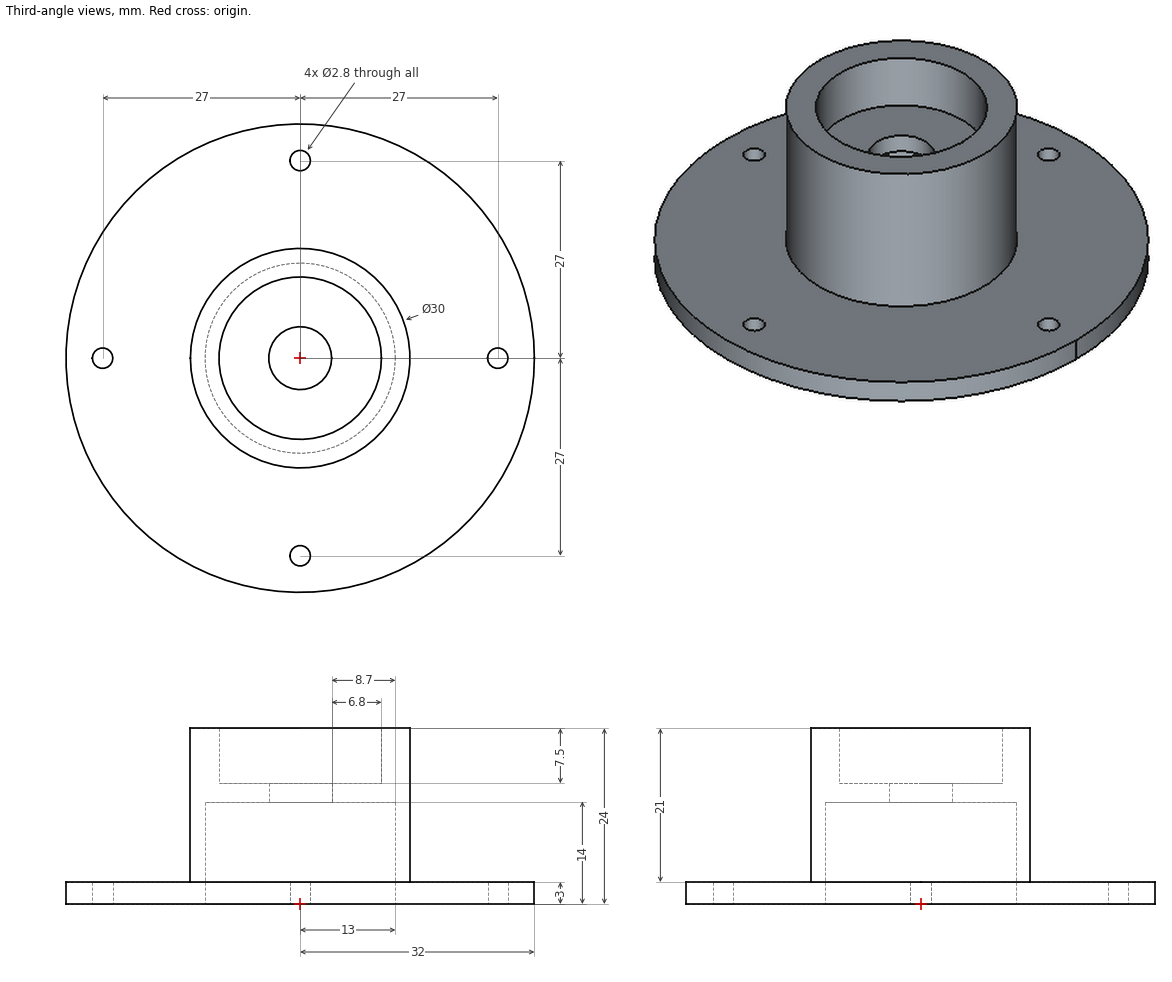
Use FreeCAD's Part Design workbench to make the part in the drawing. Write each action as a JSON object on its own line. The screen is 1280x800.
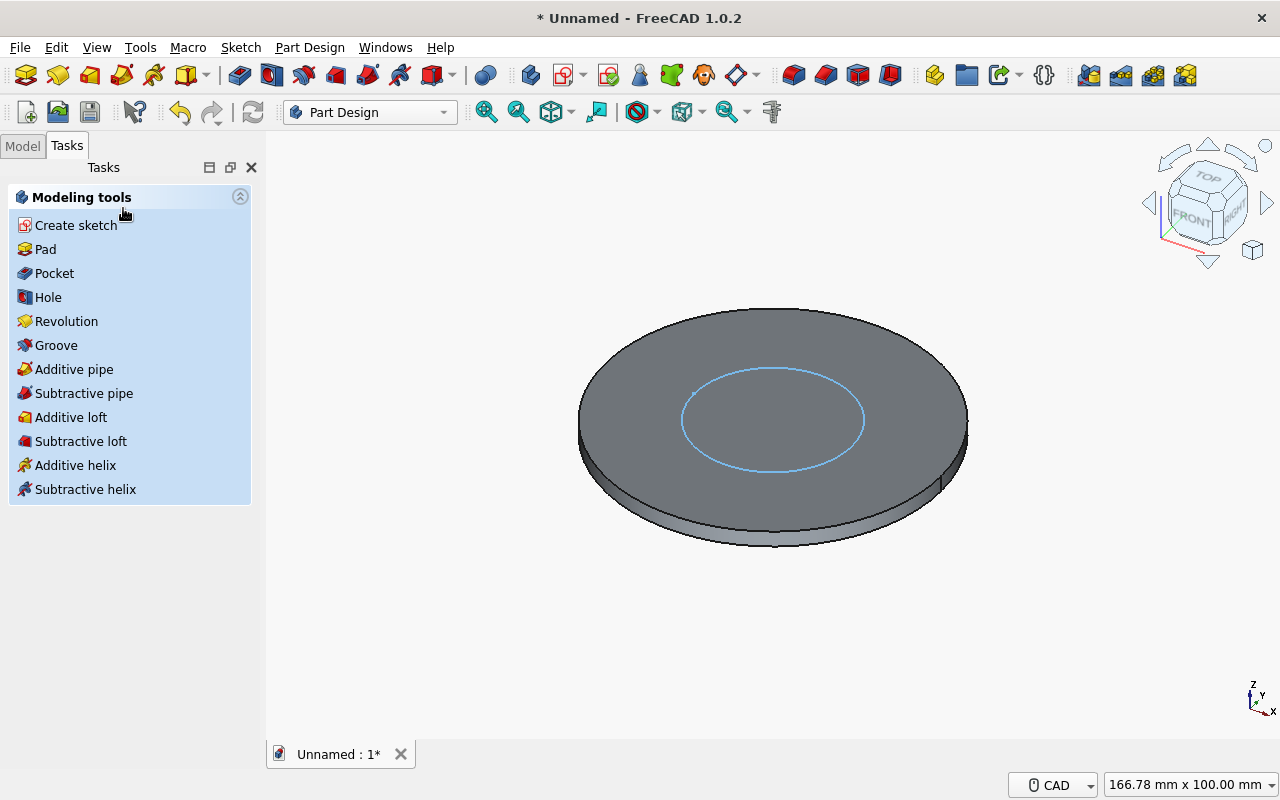
{"action": "left_click", "coordinate": [26, 76]}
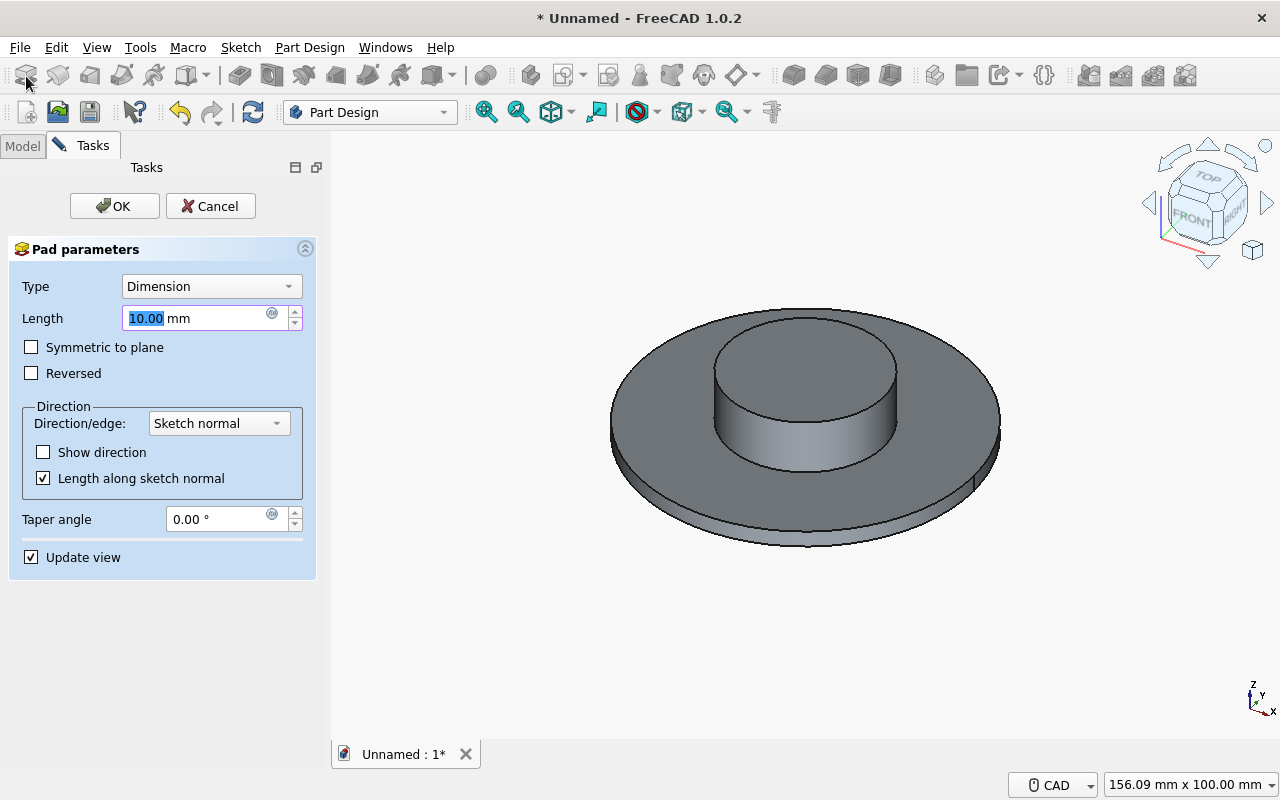
{"action": "type", "text": "21"}
{"action": "key", "text": "Tab"}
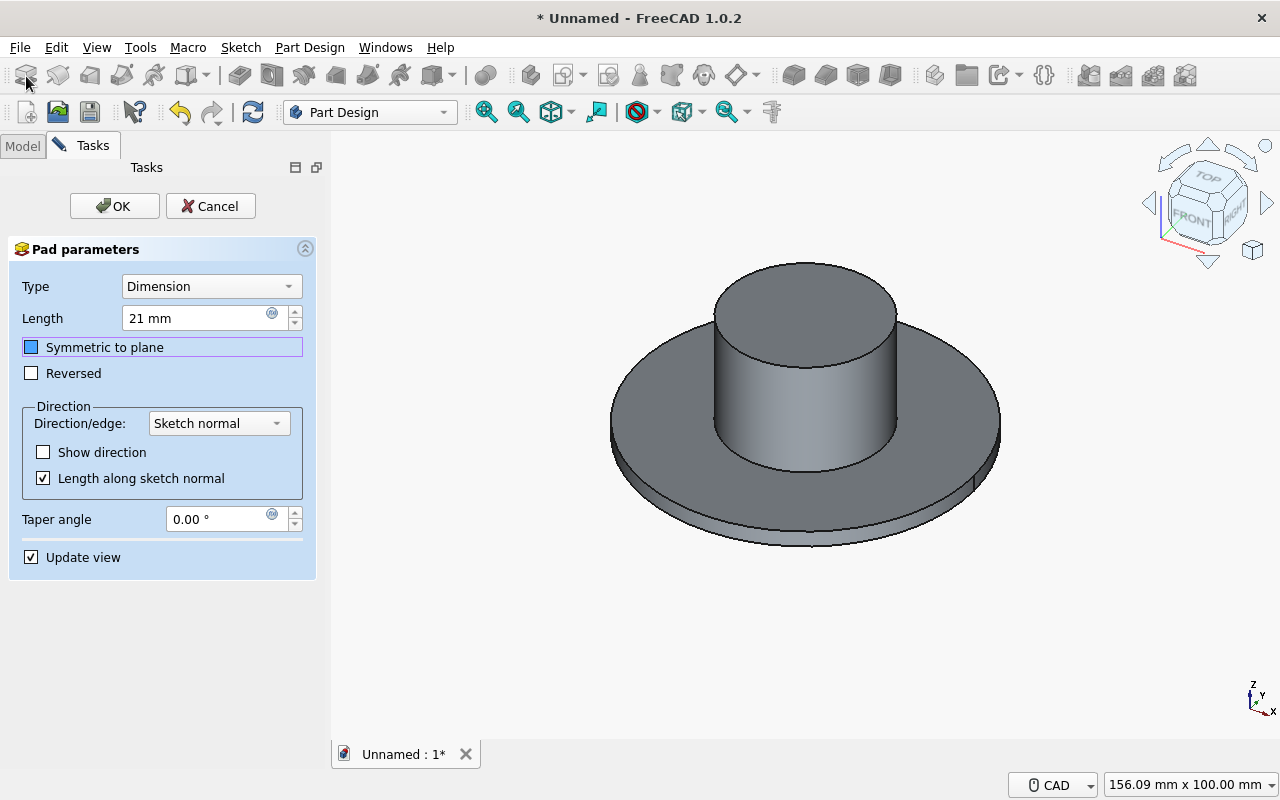
{"action": "left_click", "coordinate": [115, 206]}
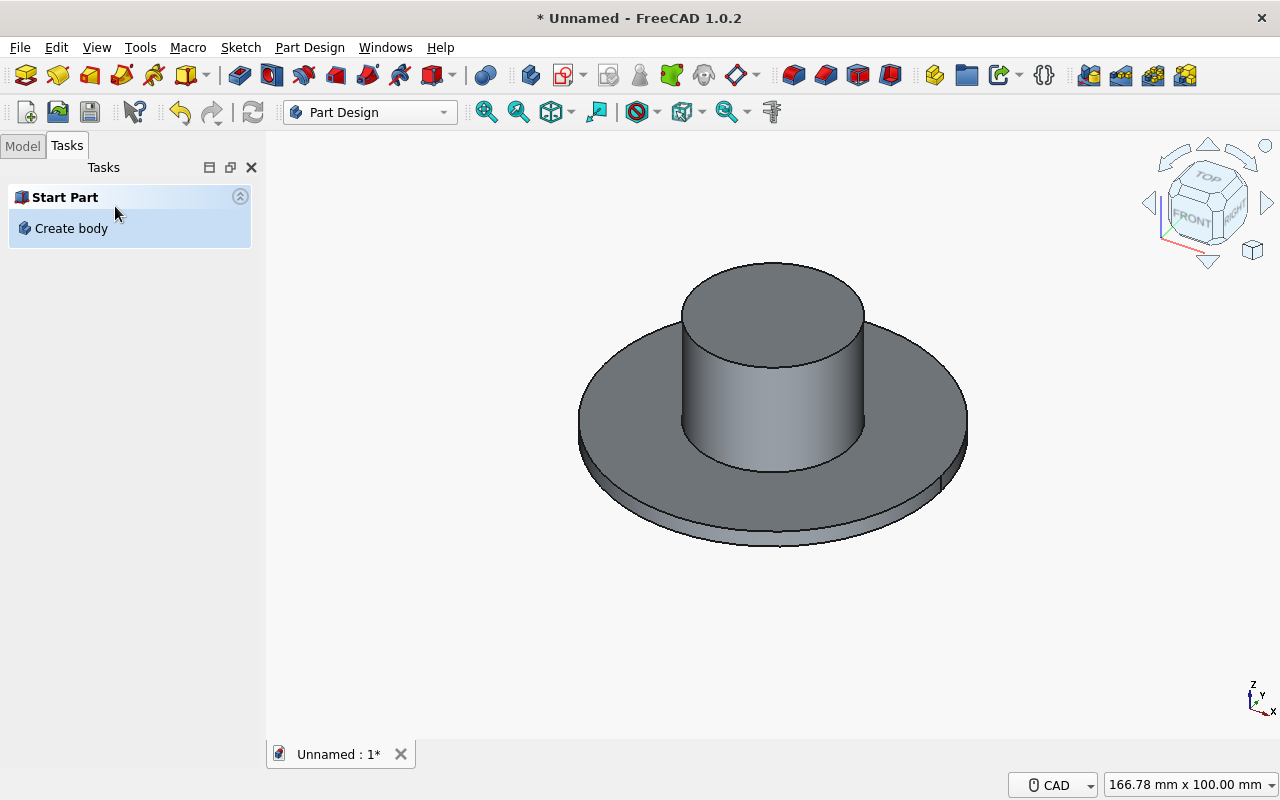
{"action": "left_click", "coordinate": [564, 76]}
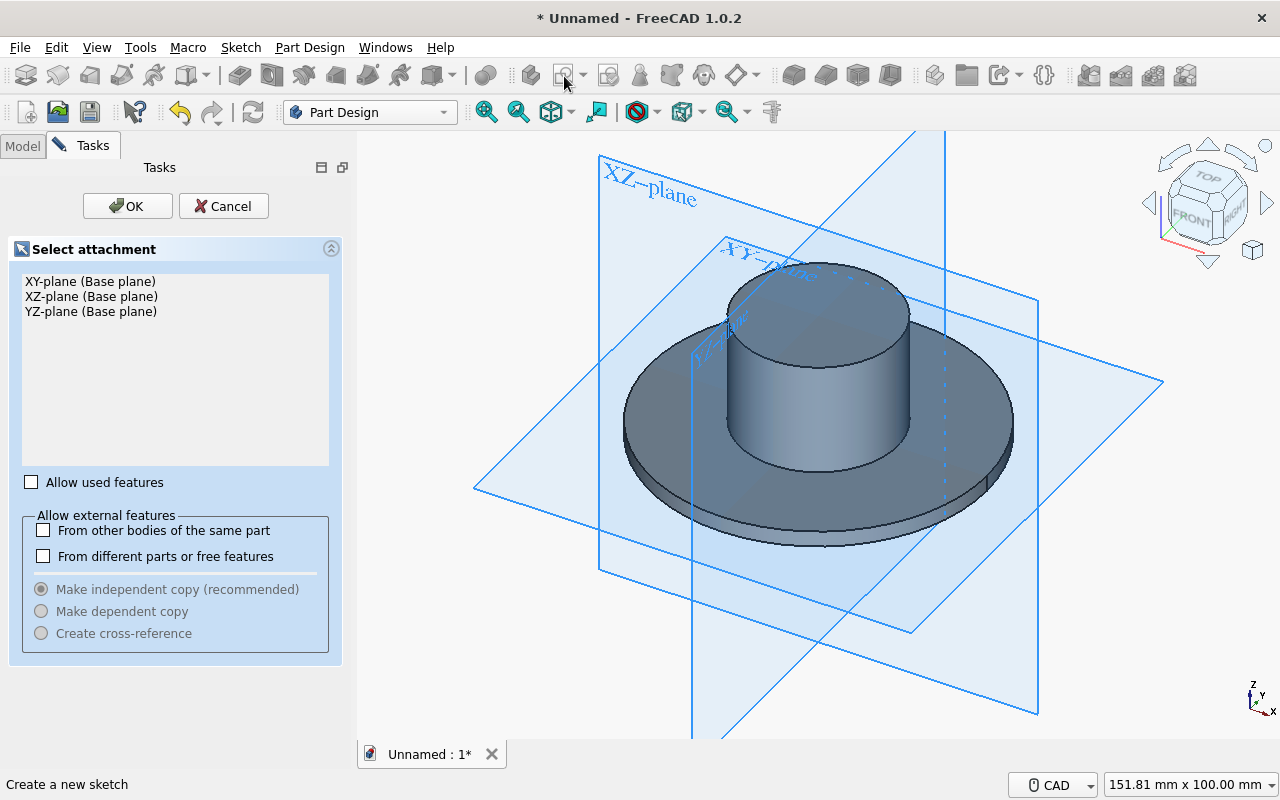
{"action": "left_click", "coordinate": [82, 296]}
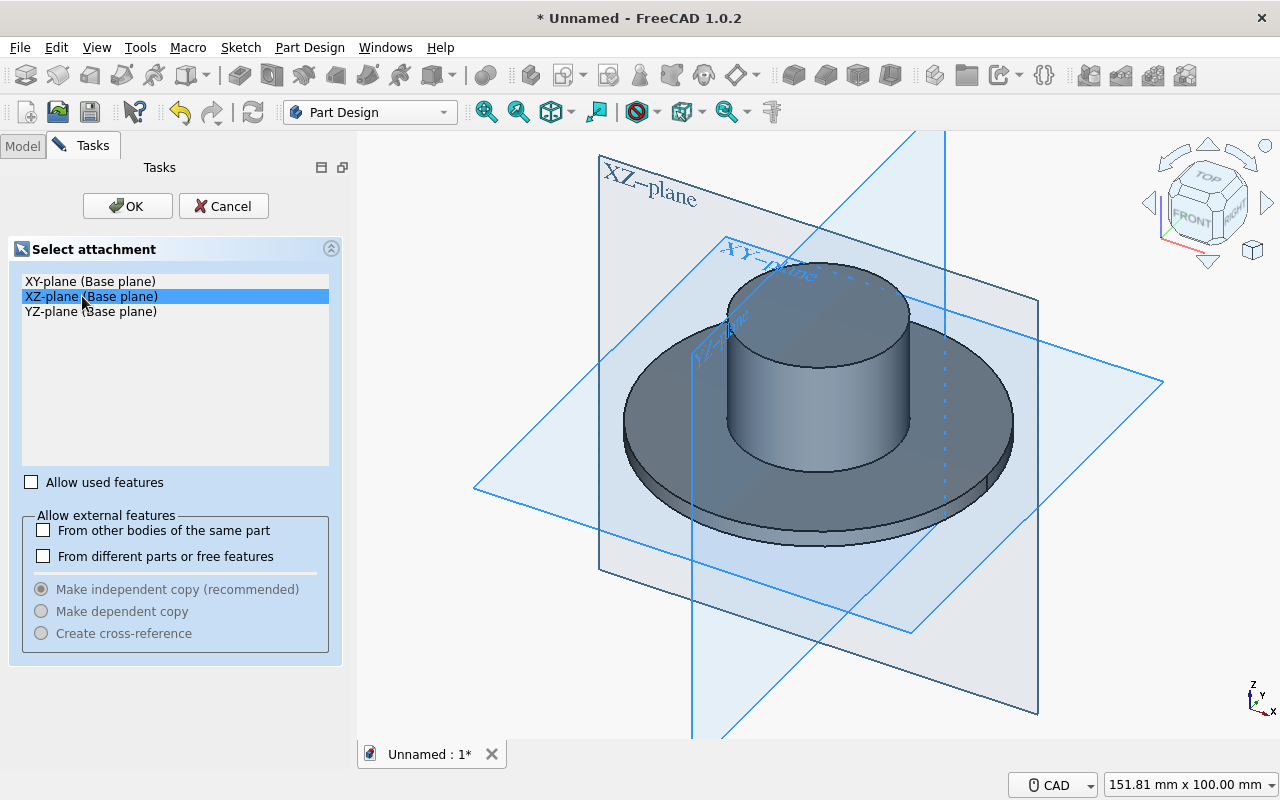
{"action": "left_click", "coordinate": [128, 206]}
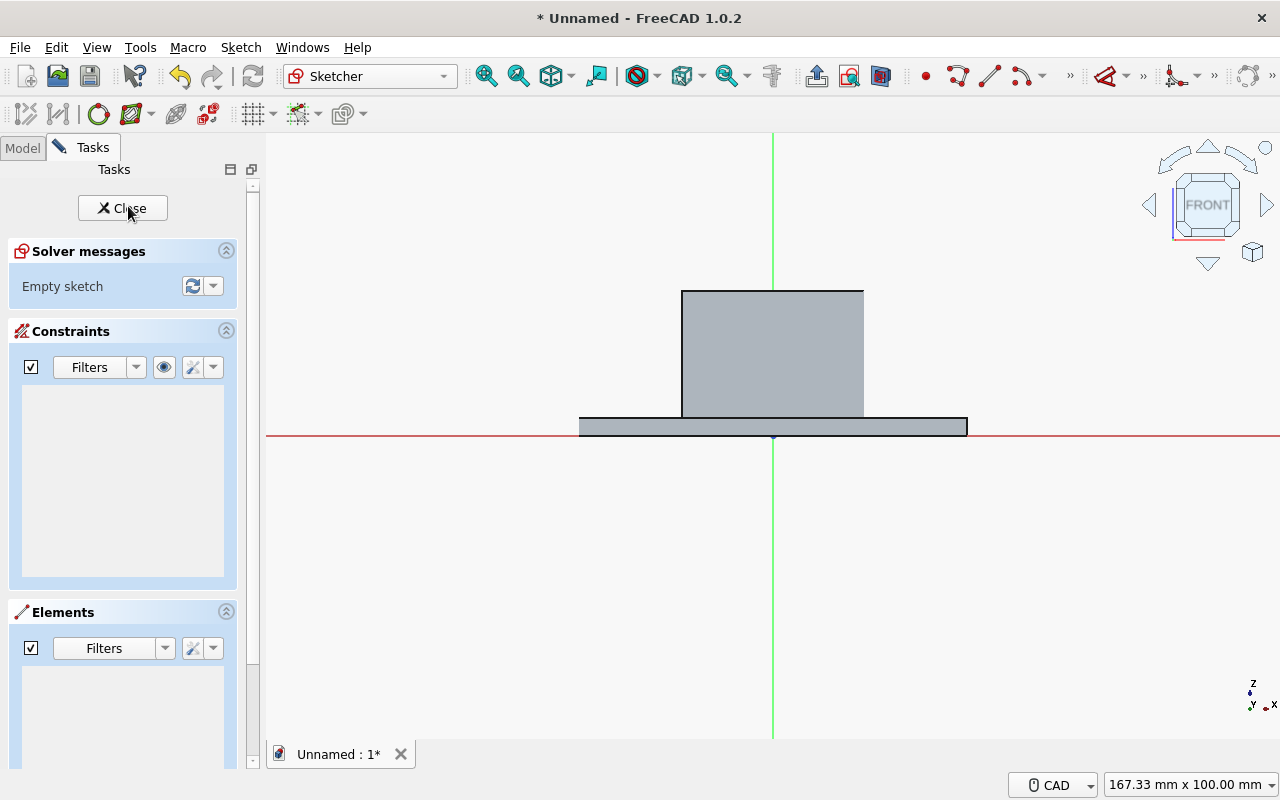
{"action": "left_click", "coordinate": [882, 76]}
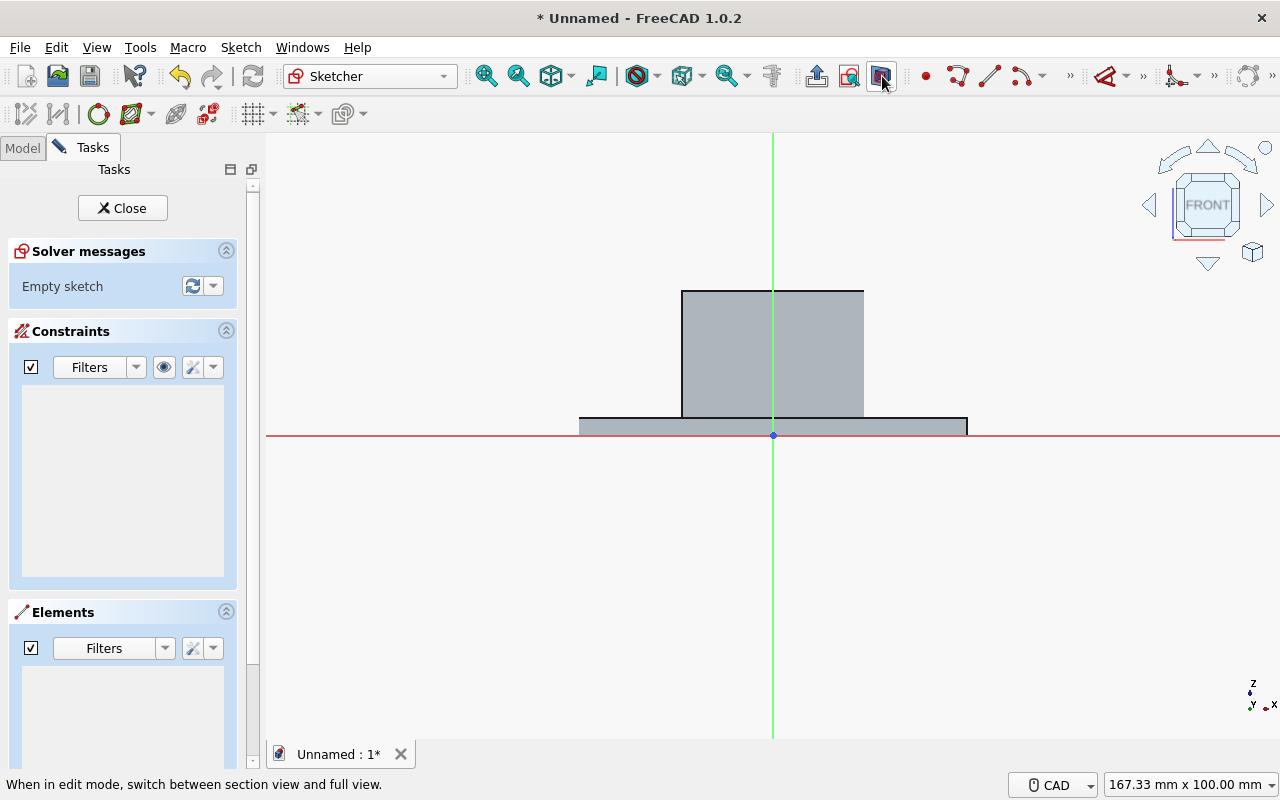
{"action": "scroll", "coordinate": [875, 321], "scroll_direction": "up", "scroll_amount": 5}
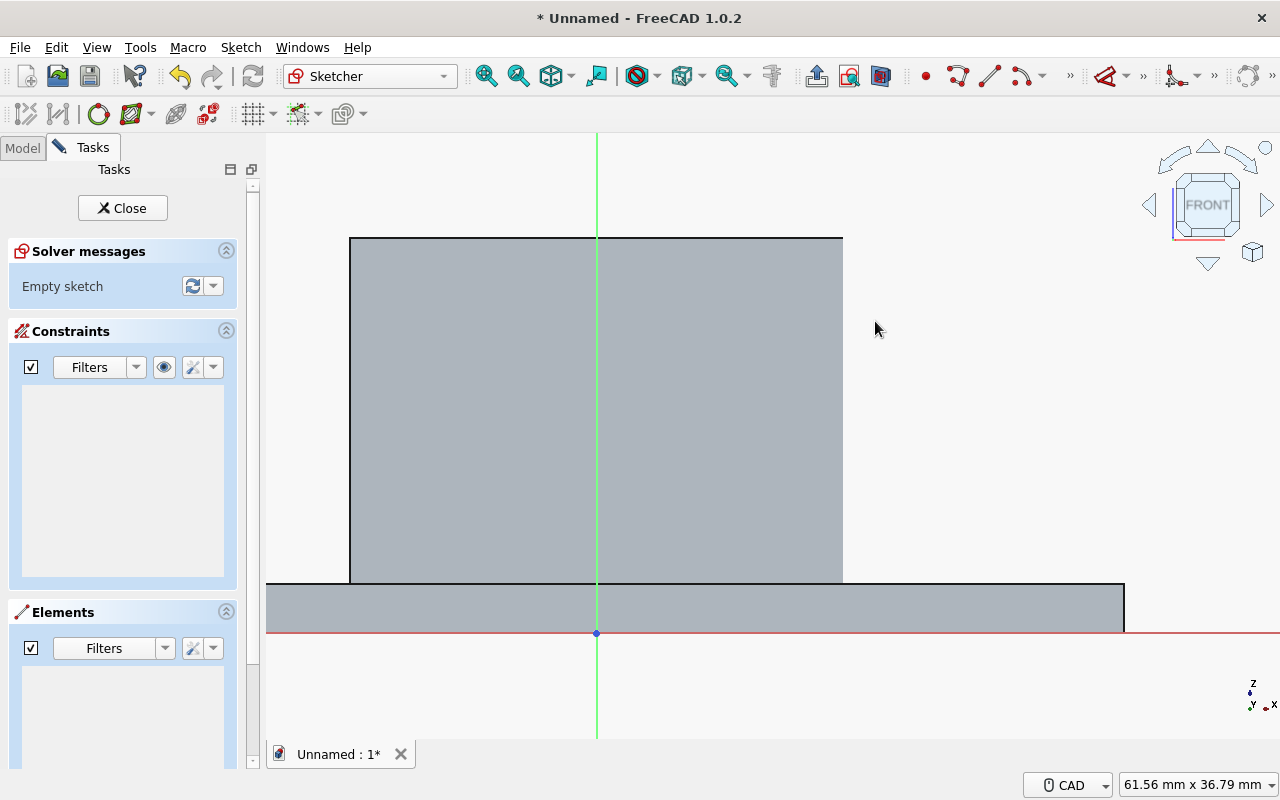
{"action": "left_click", "coordinate": [958, 76]}